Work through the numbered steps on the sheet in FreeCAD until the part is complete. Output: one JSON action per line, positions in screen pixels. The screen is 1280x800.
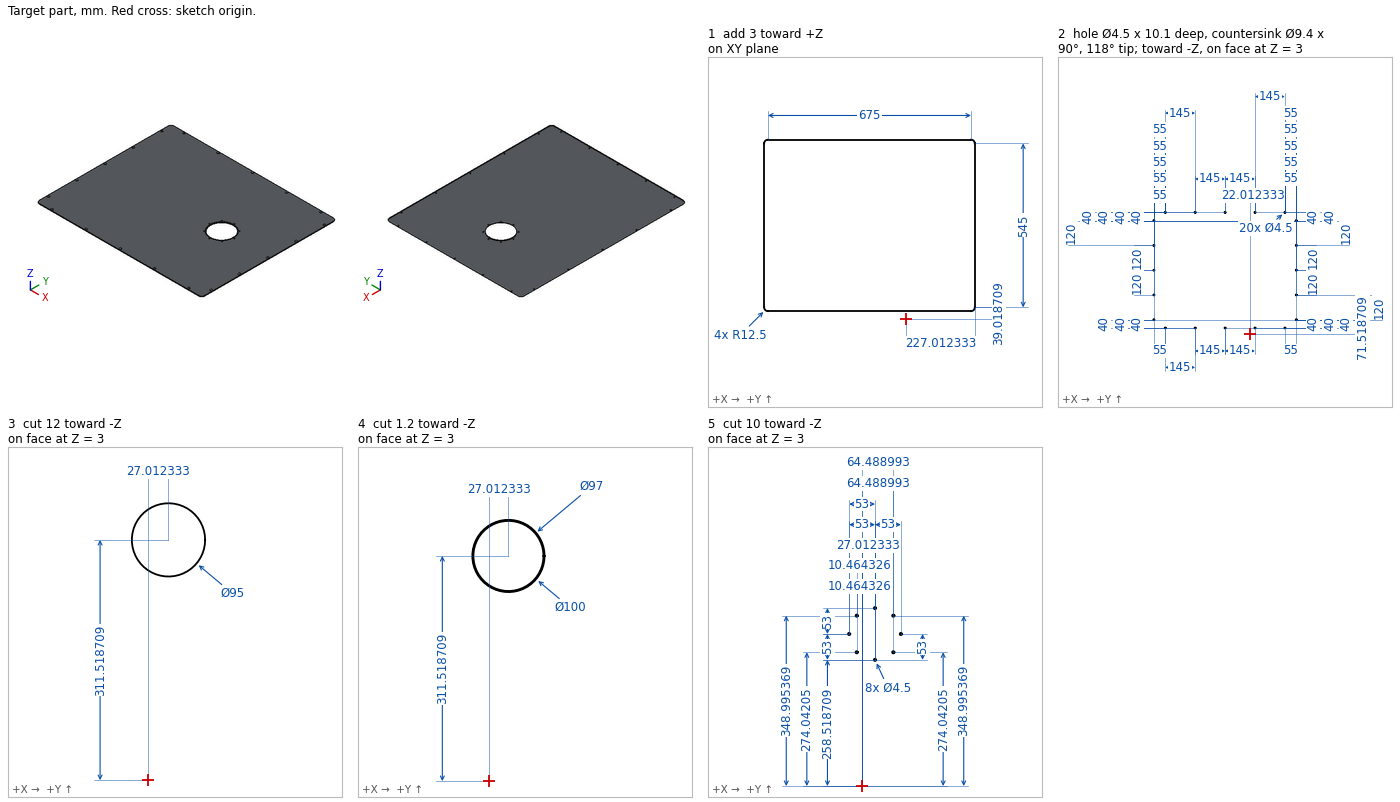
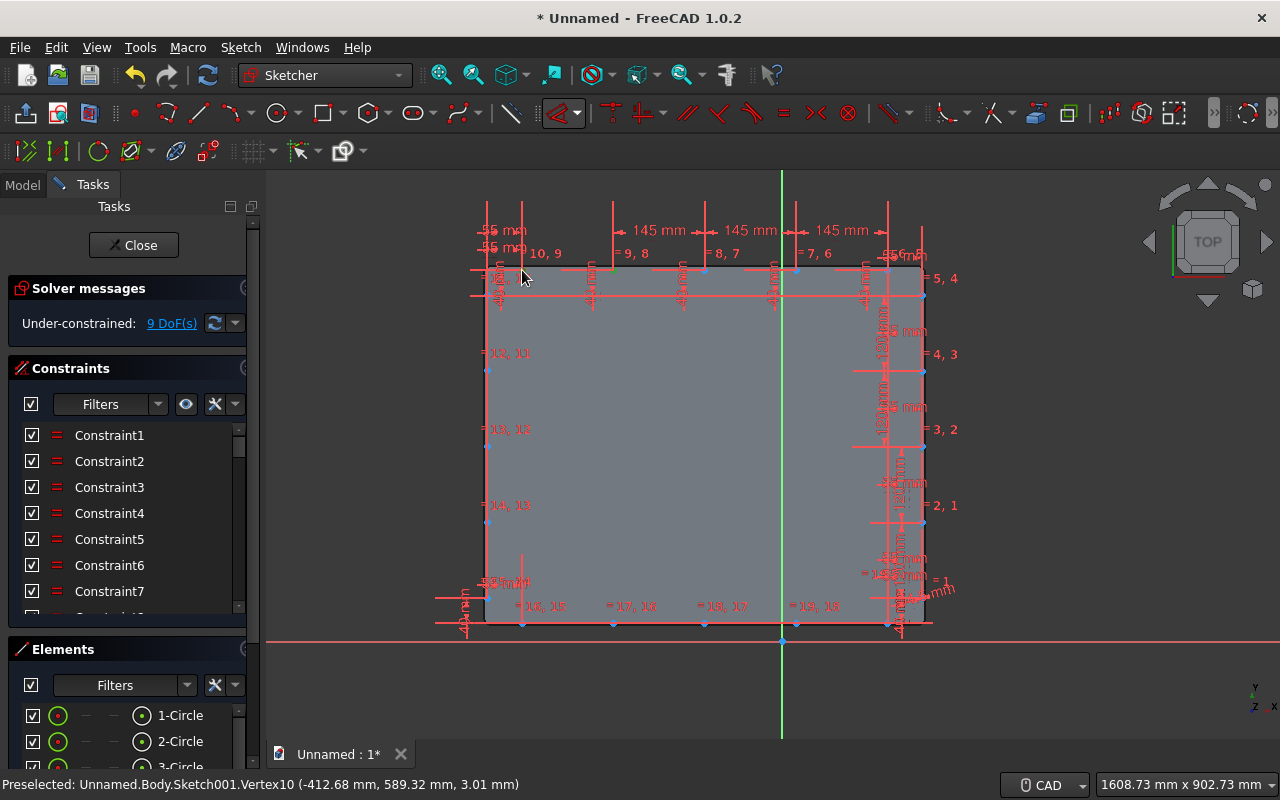
{"action": "key", "text": "l"}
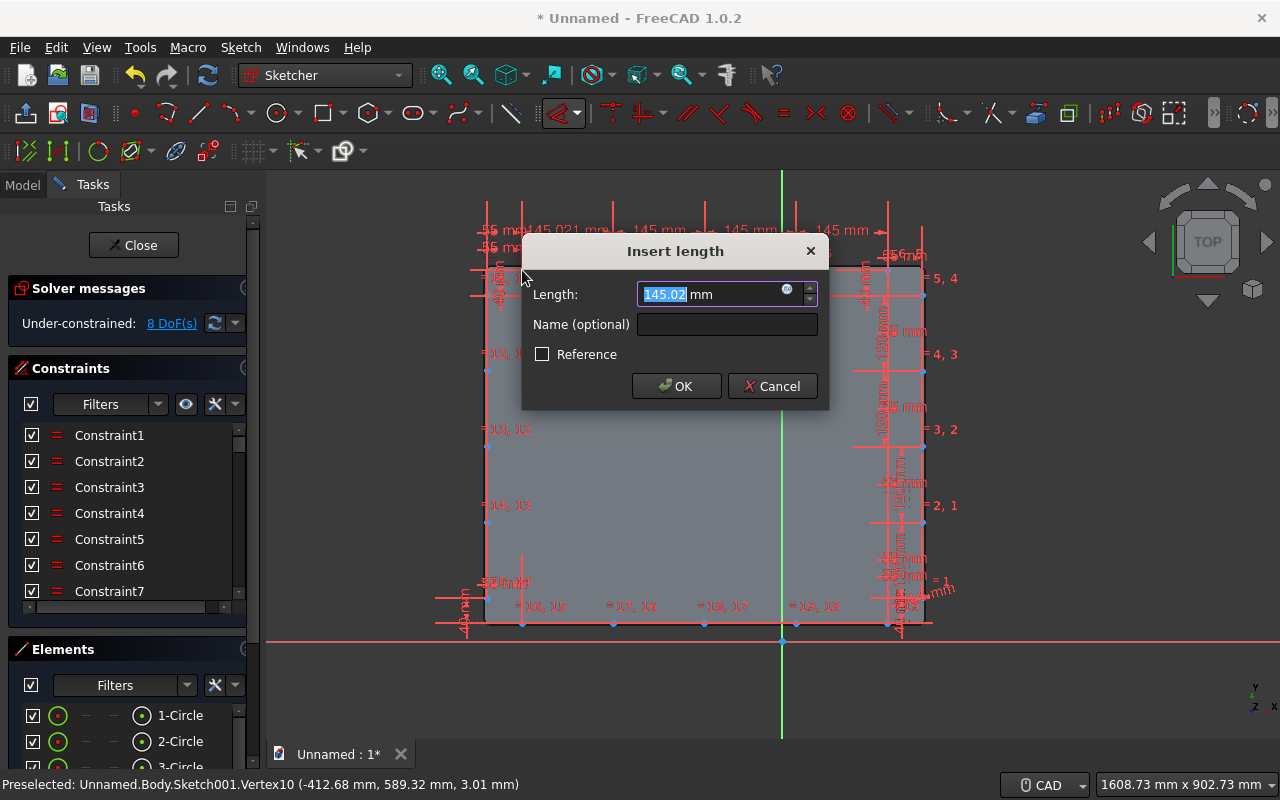
{"action": "type", "text": "145"}
{"action": "key", "text": "Return"}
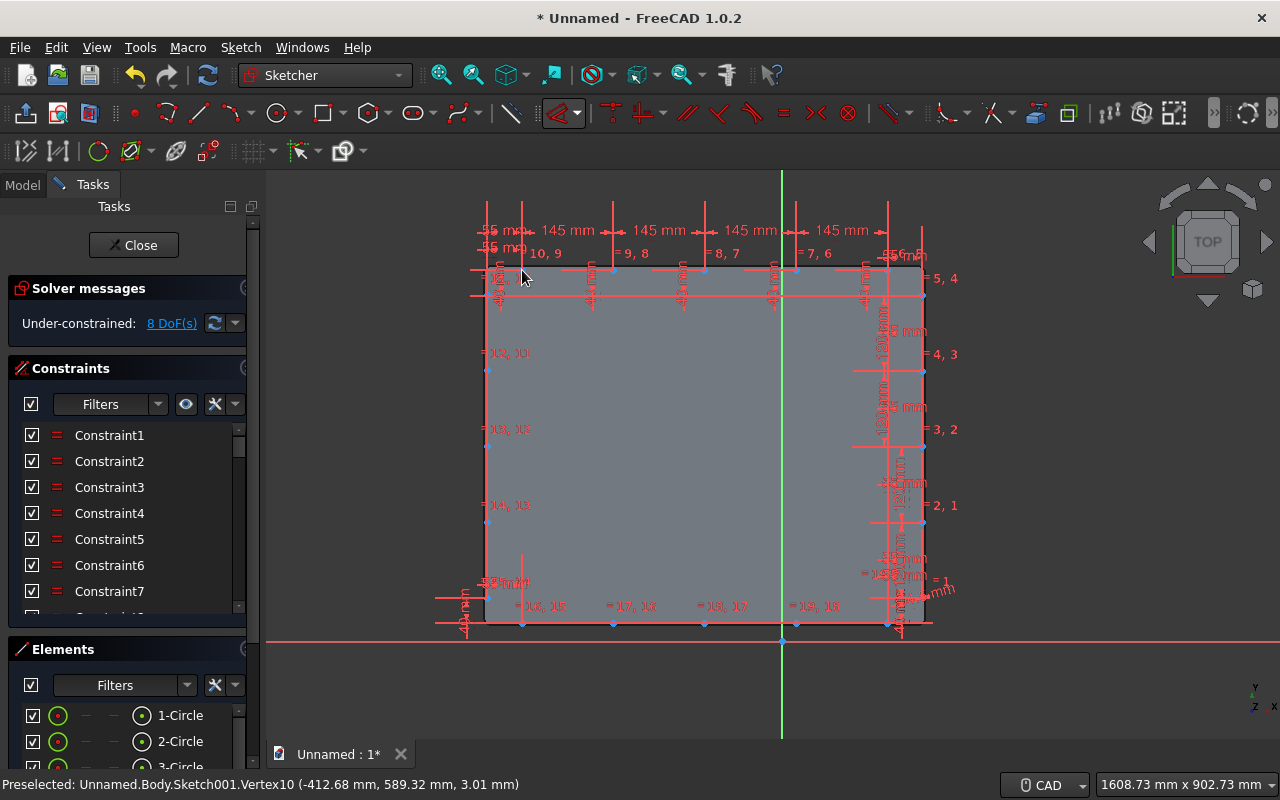
{"action": "left_click", "coordinate": [487, 296]}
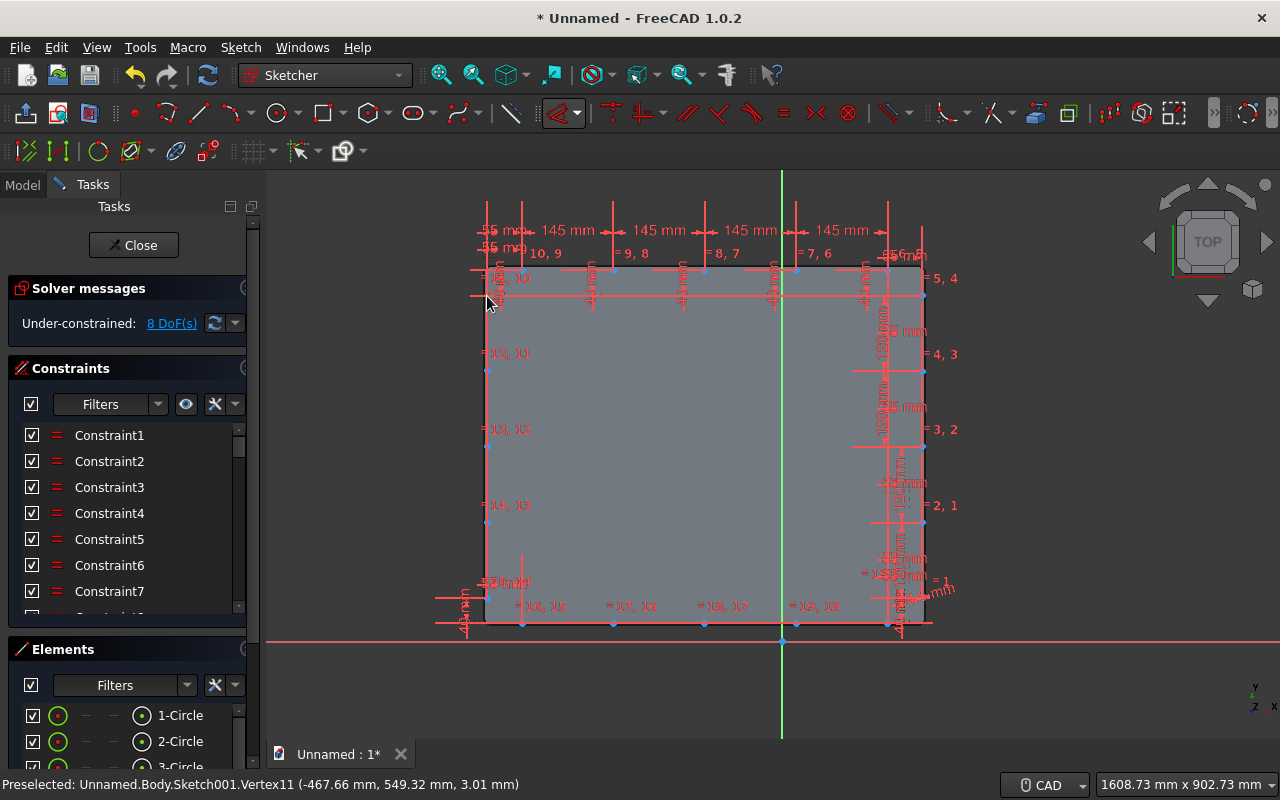
{"action": "left_click", "coordinate": [487, 370]}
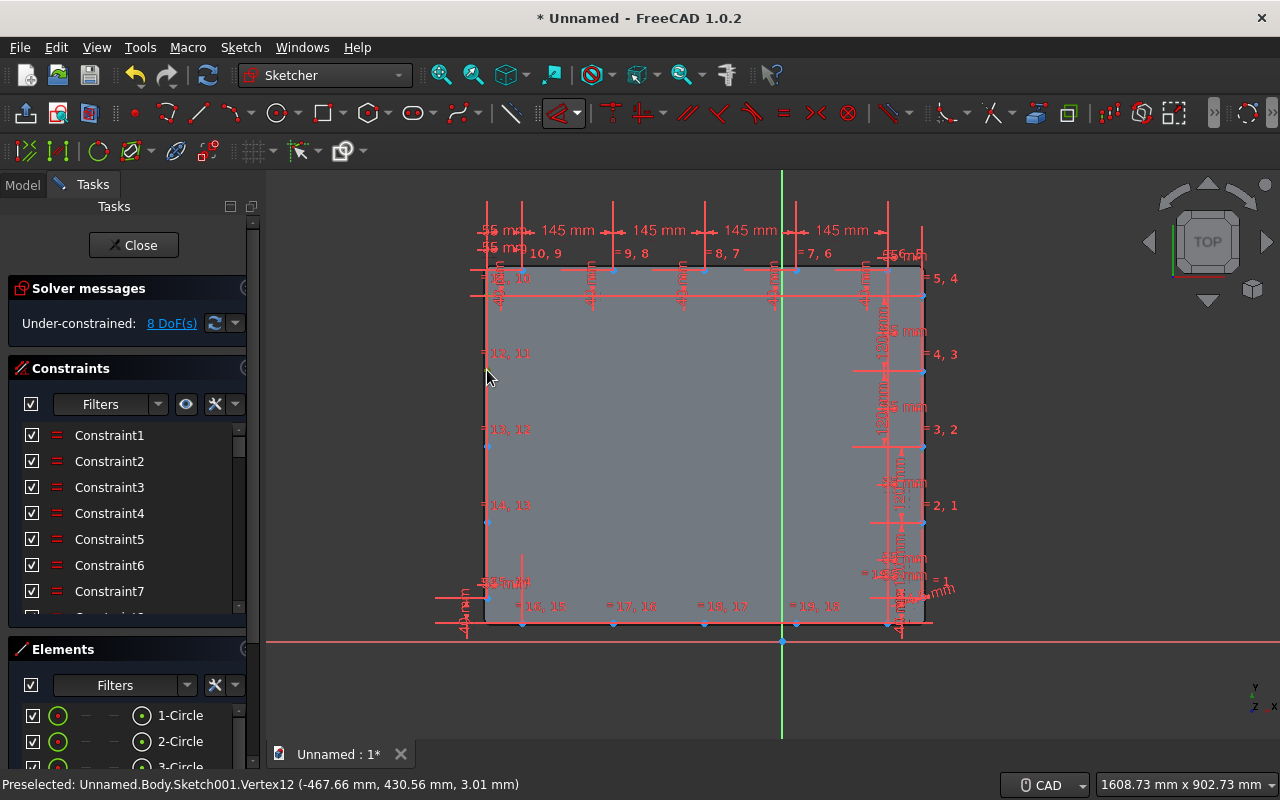
{"action": "key", "text": "i"}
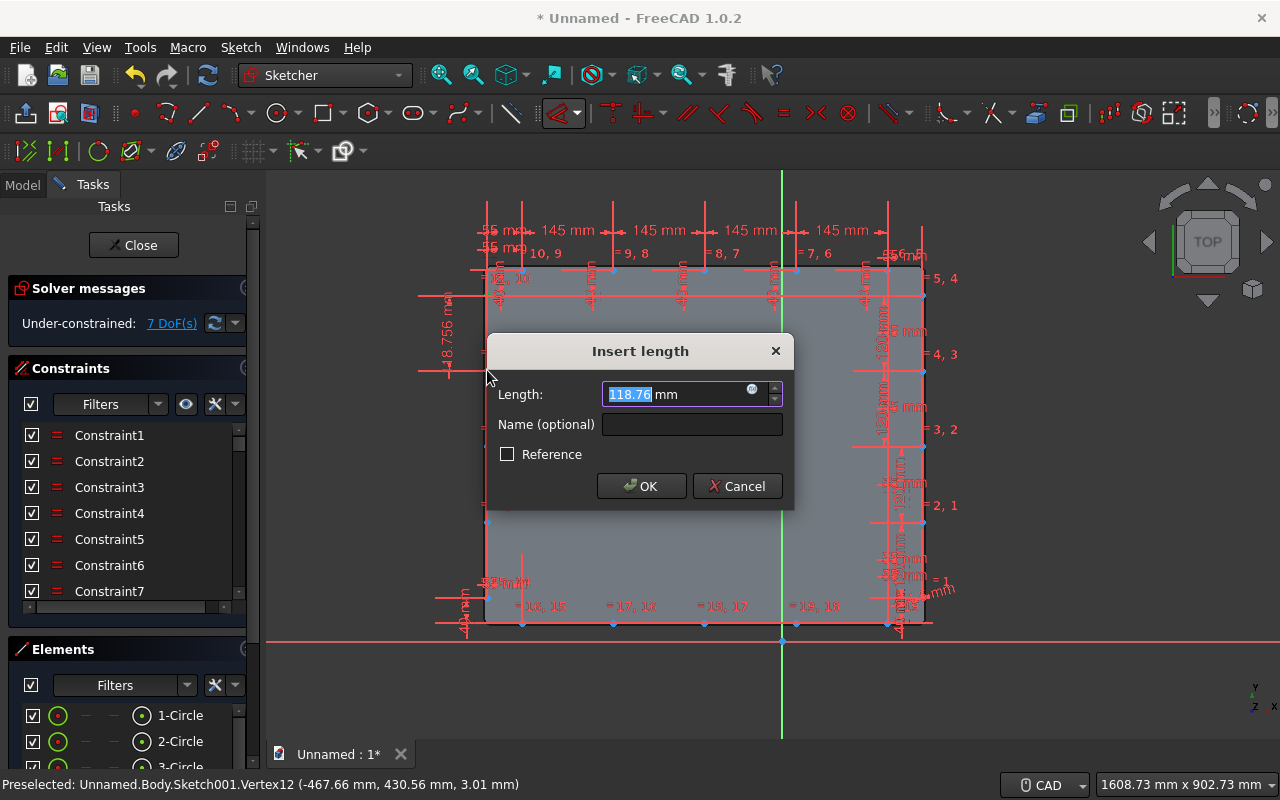
{"action": "type", "text": "120"}
{"action": "key", "text": "Return"}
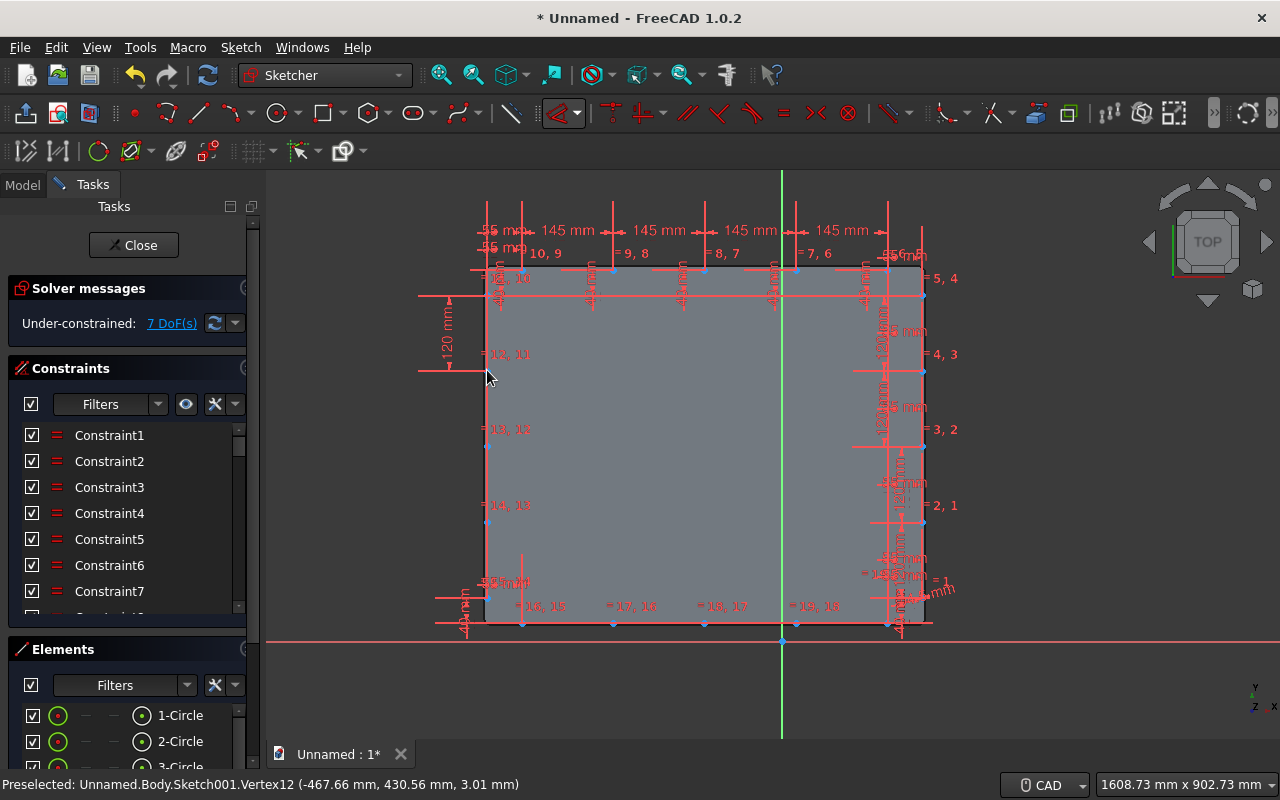
{"action": "left_click", "coordinate": [487, 371]}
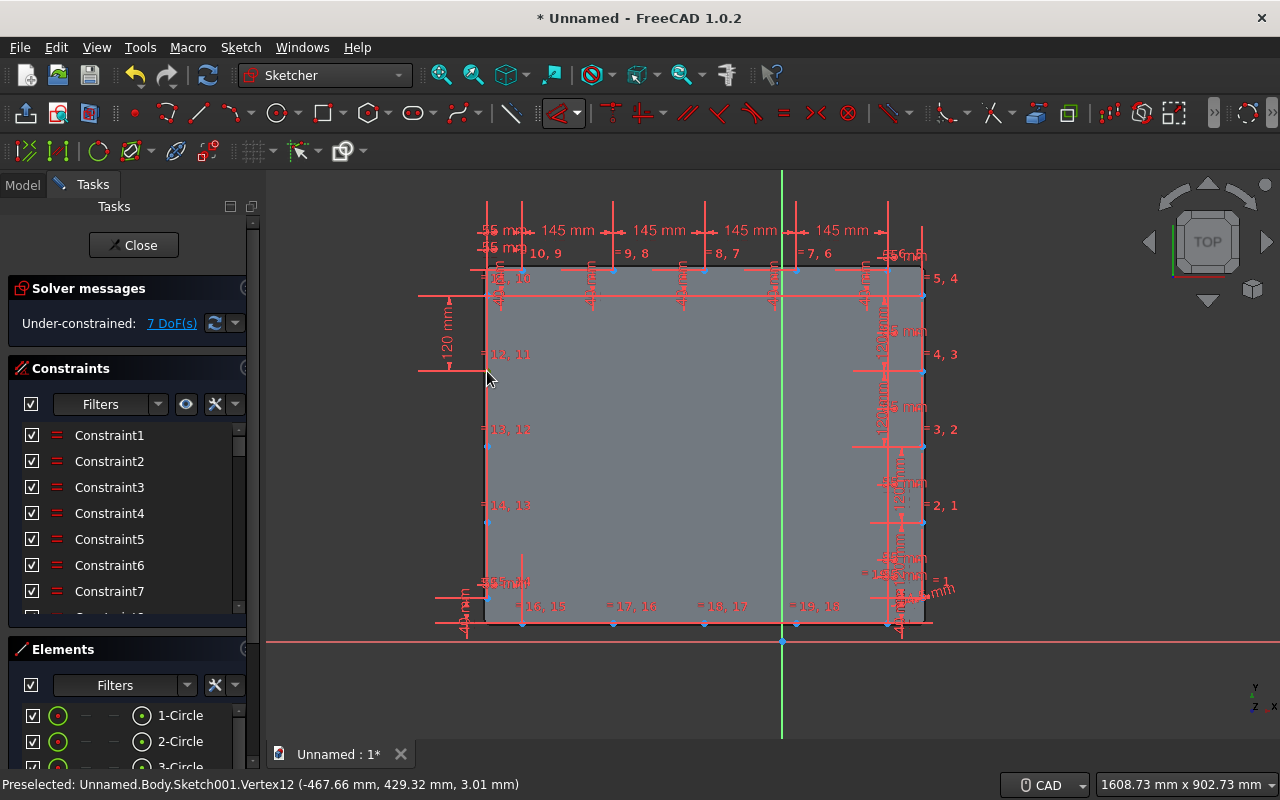
{"action": "left_click", "coordinate": [487, 446]}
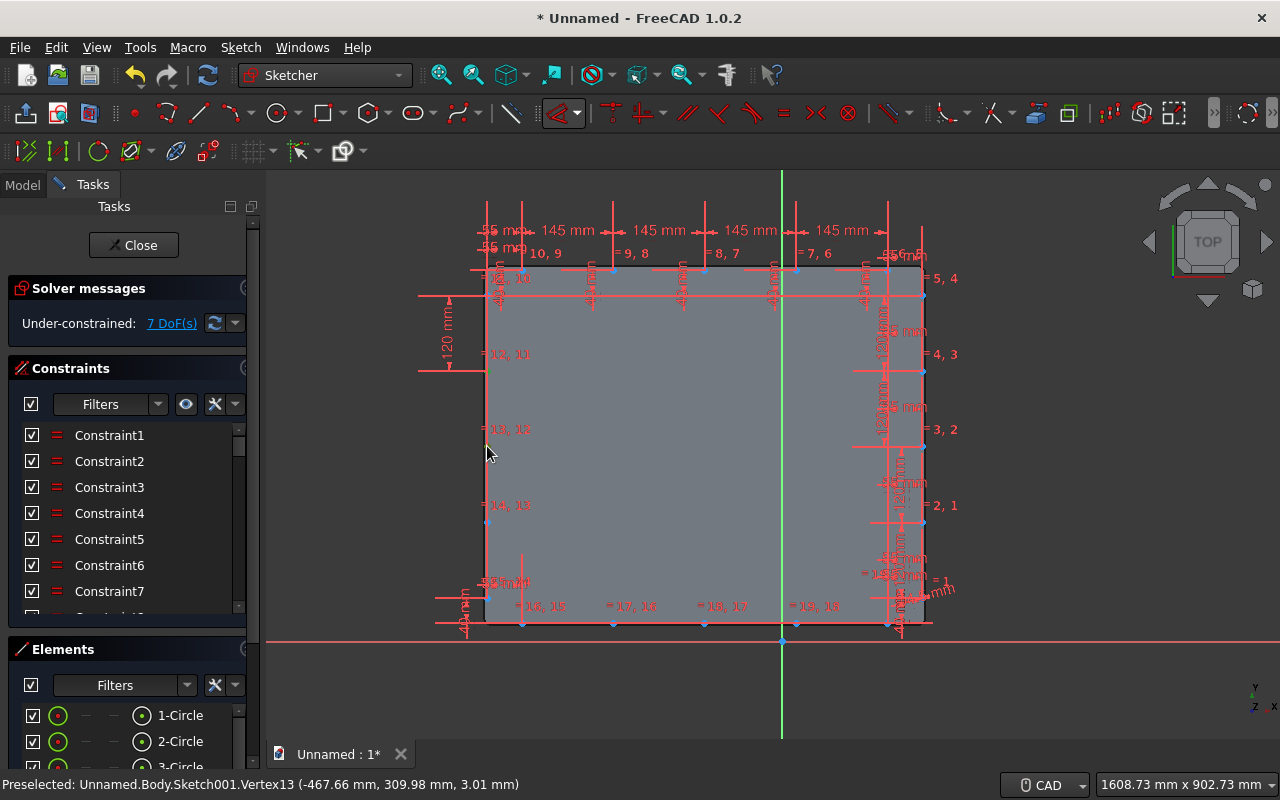
{"action": "left_click", "coordinate": [580, 114]}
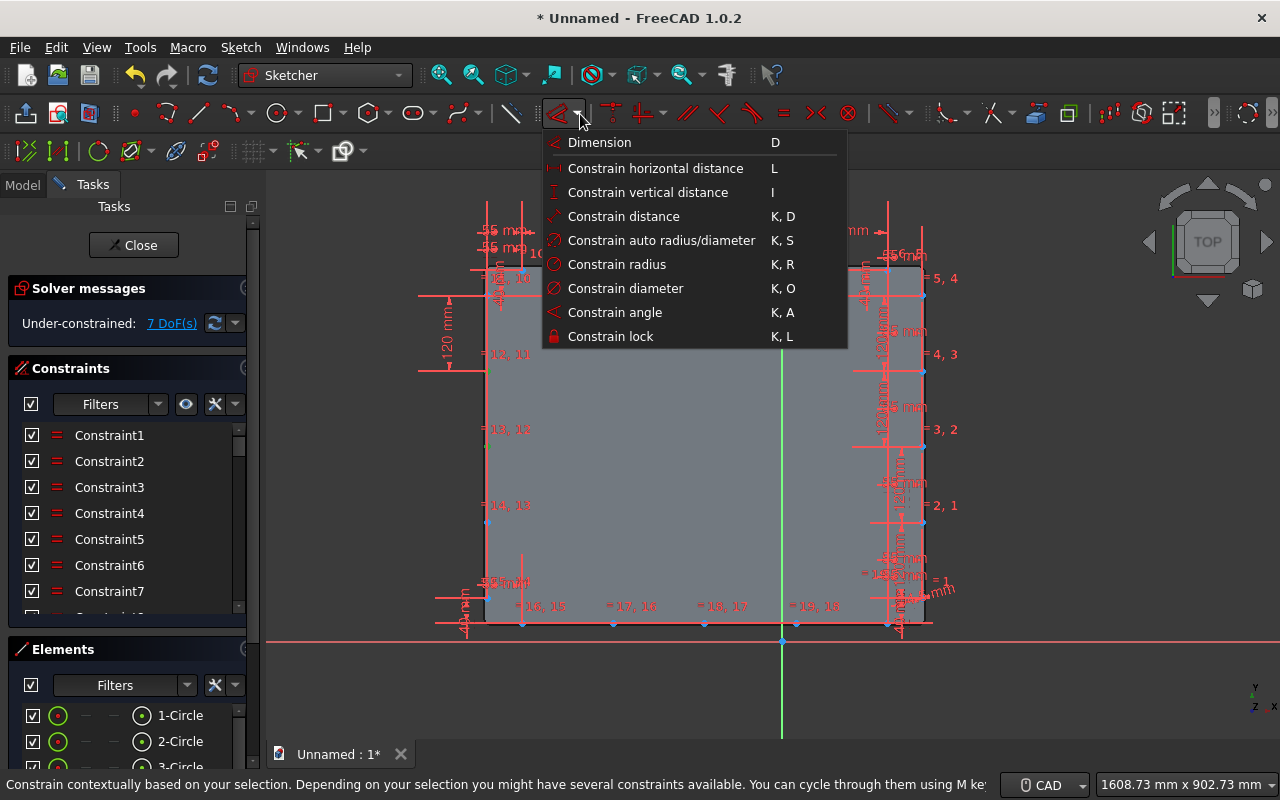
{"action": "left_click", "coordinate": [695, 192]}